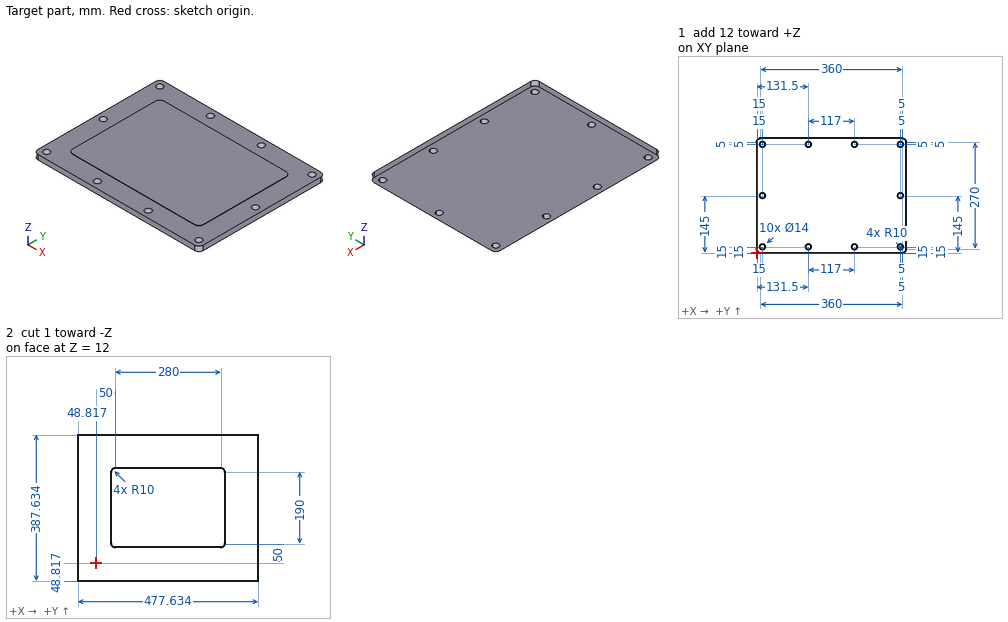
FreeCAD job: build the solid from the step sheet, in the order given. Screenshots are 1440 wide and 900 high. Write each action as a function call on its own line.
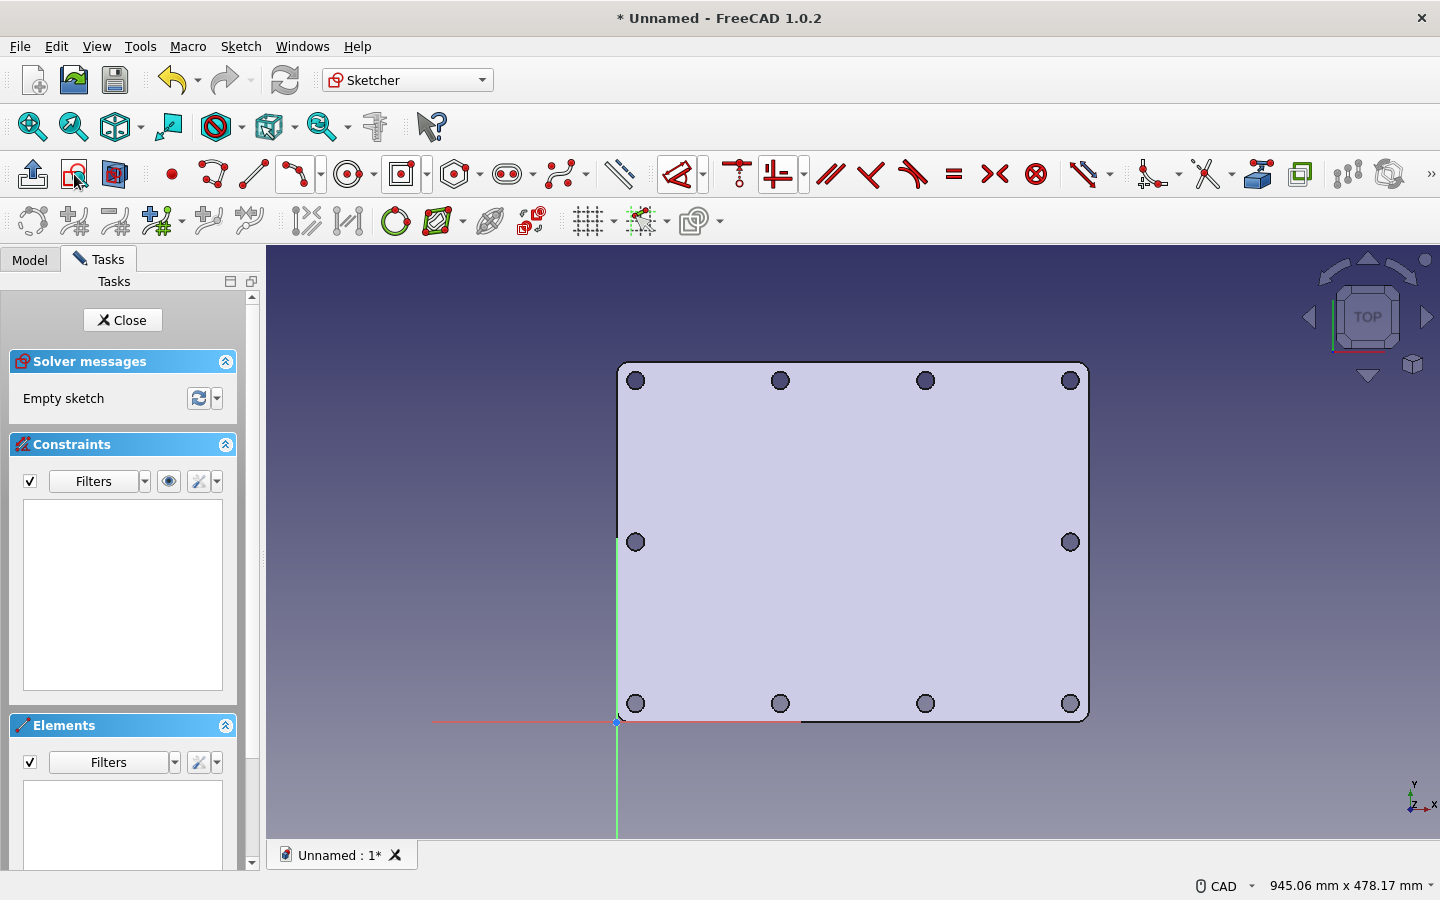
key(g)
key(r)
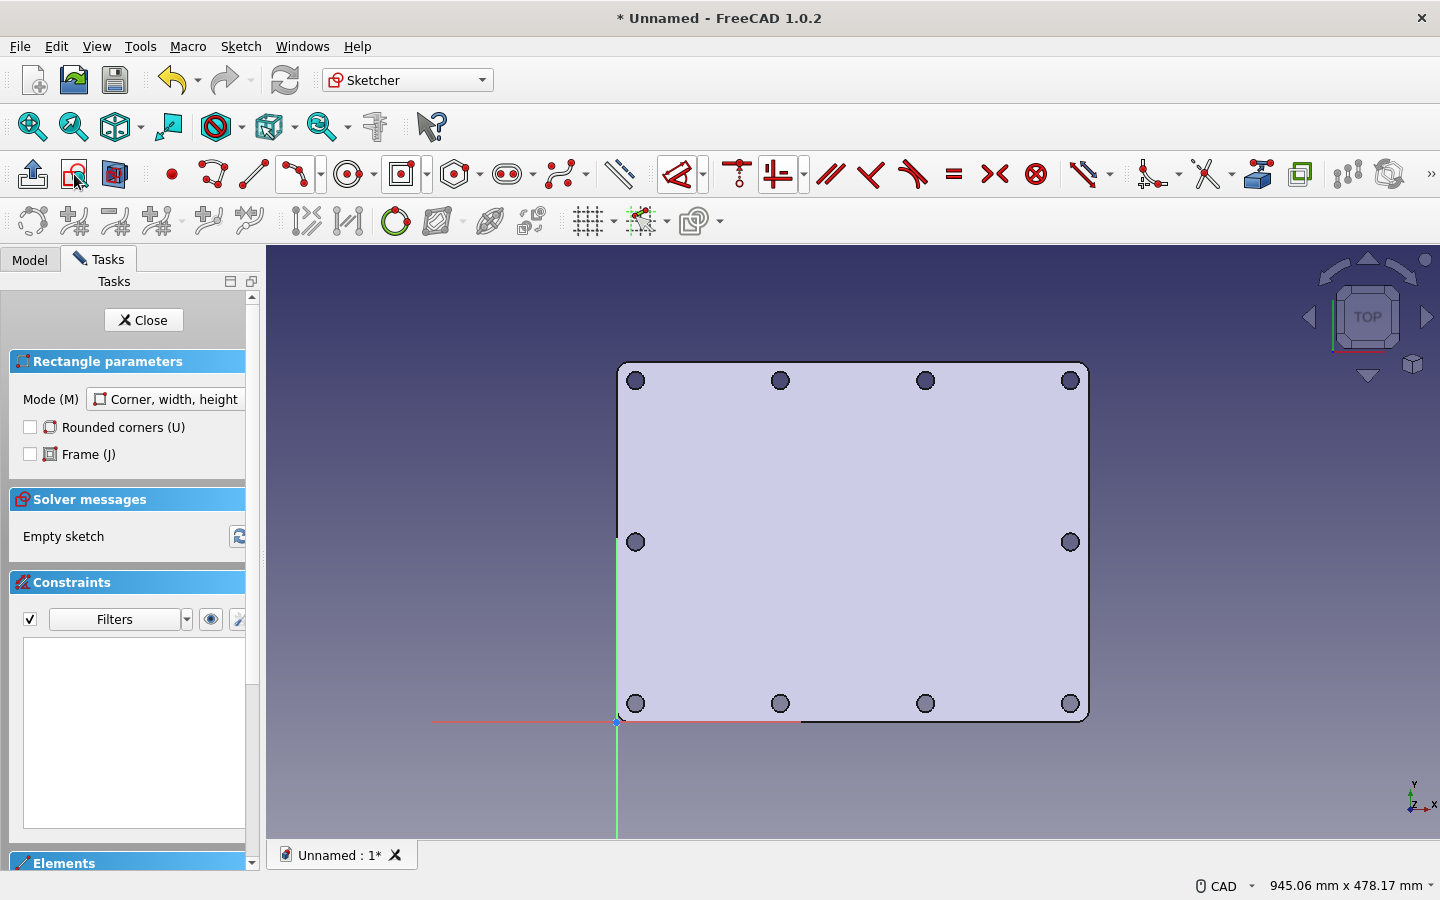
click(556, 301)
click(1150, 783)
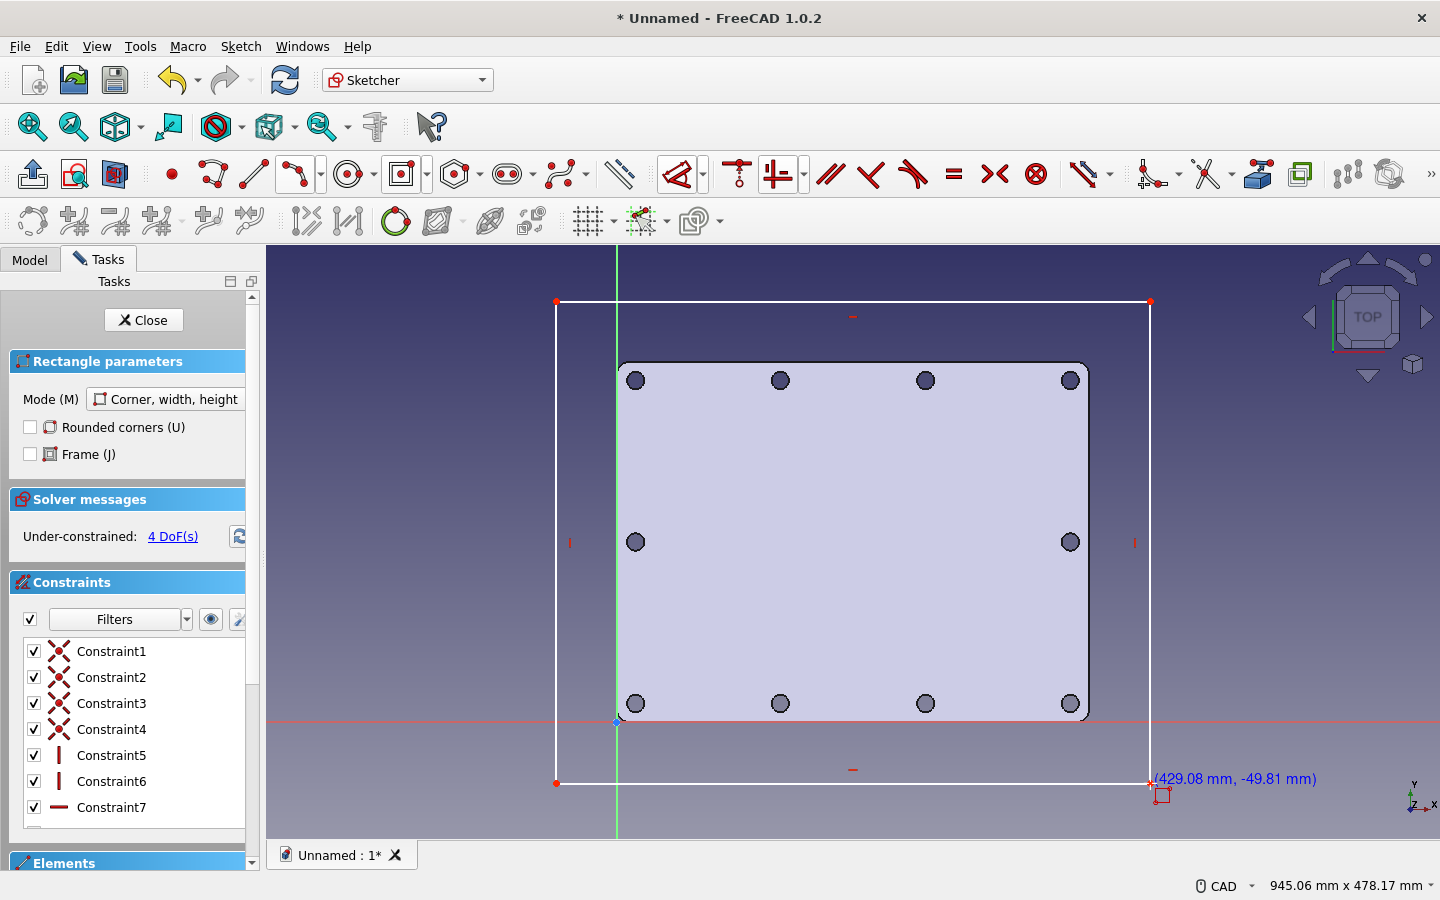
click(254, 174)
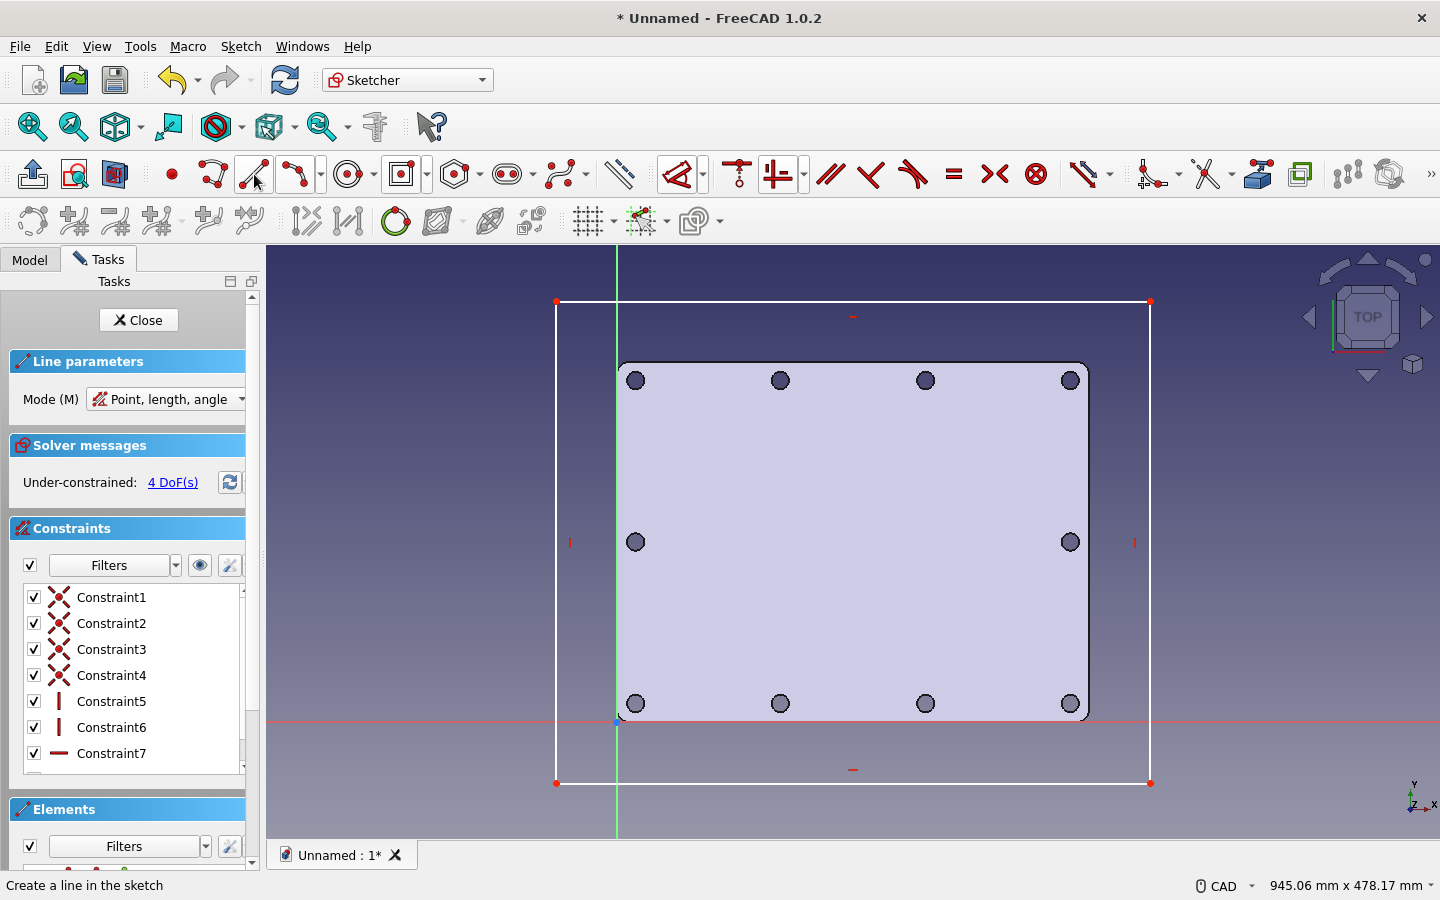
click(679, 412)
click(1027, 412)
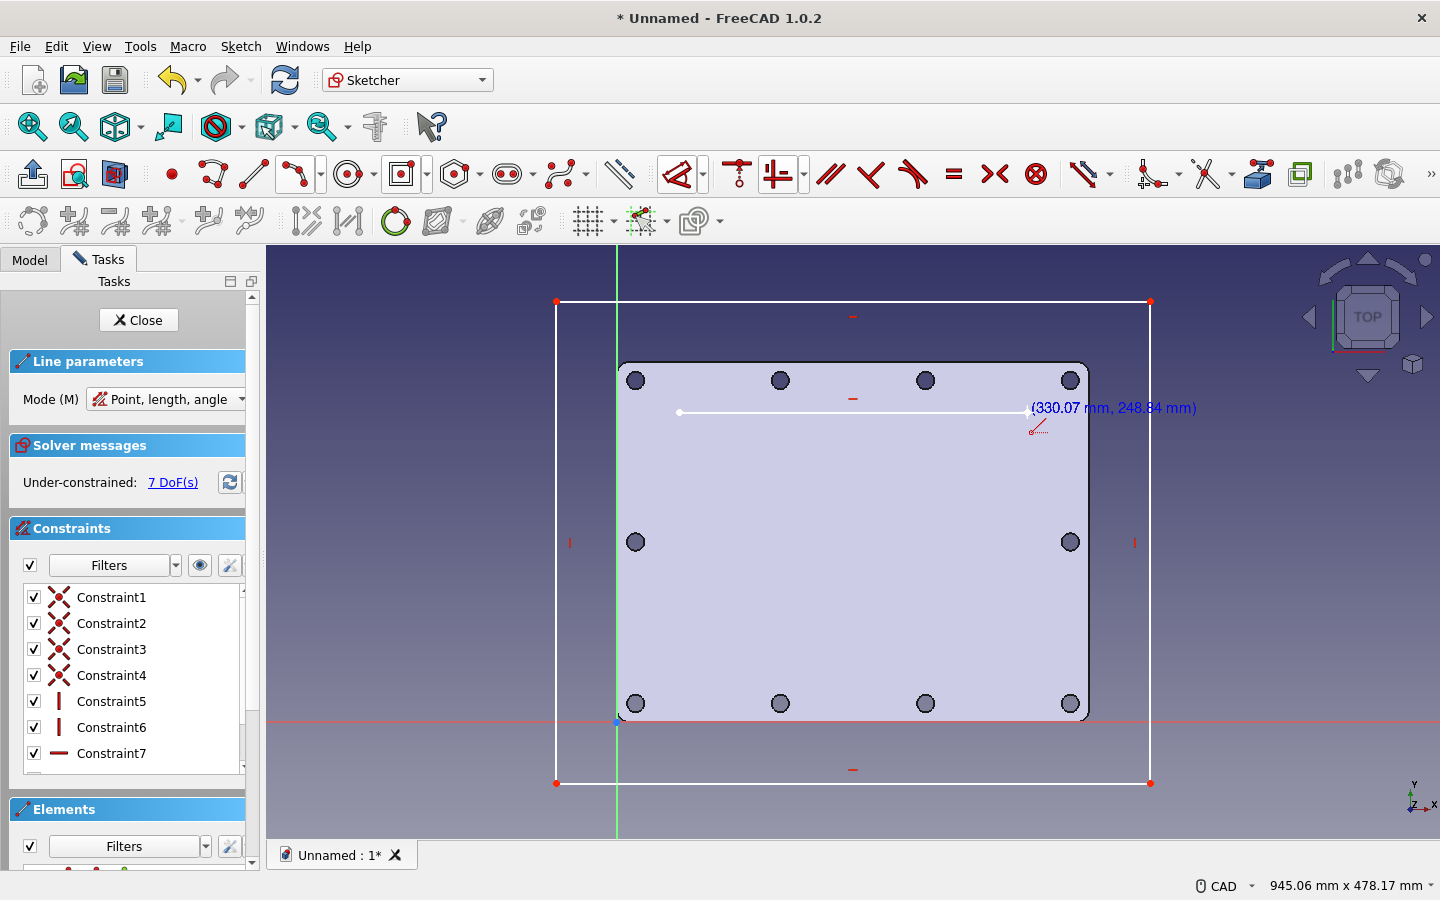
click(1039, 424)
click(1039, 660)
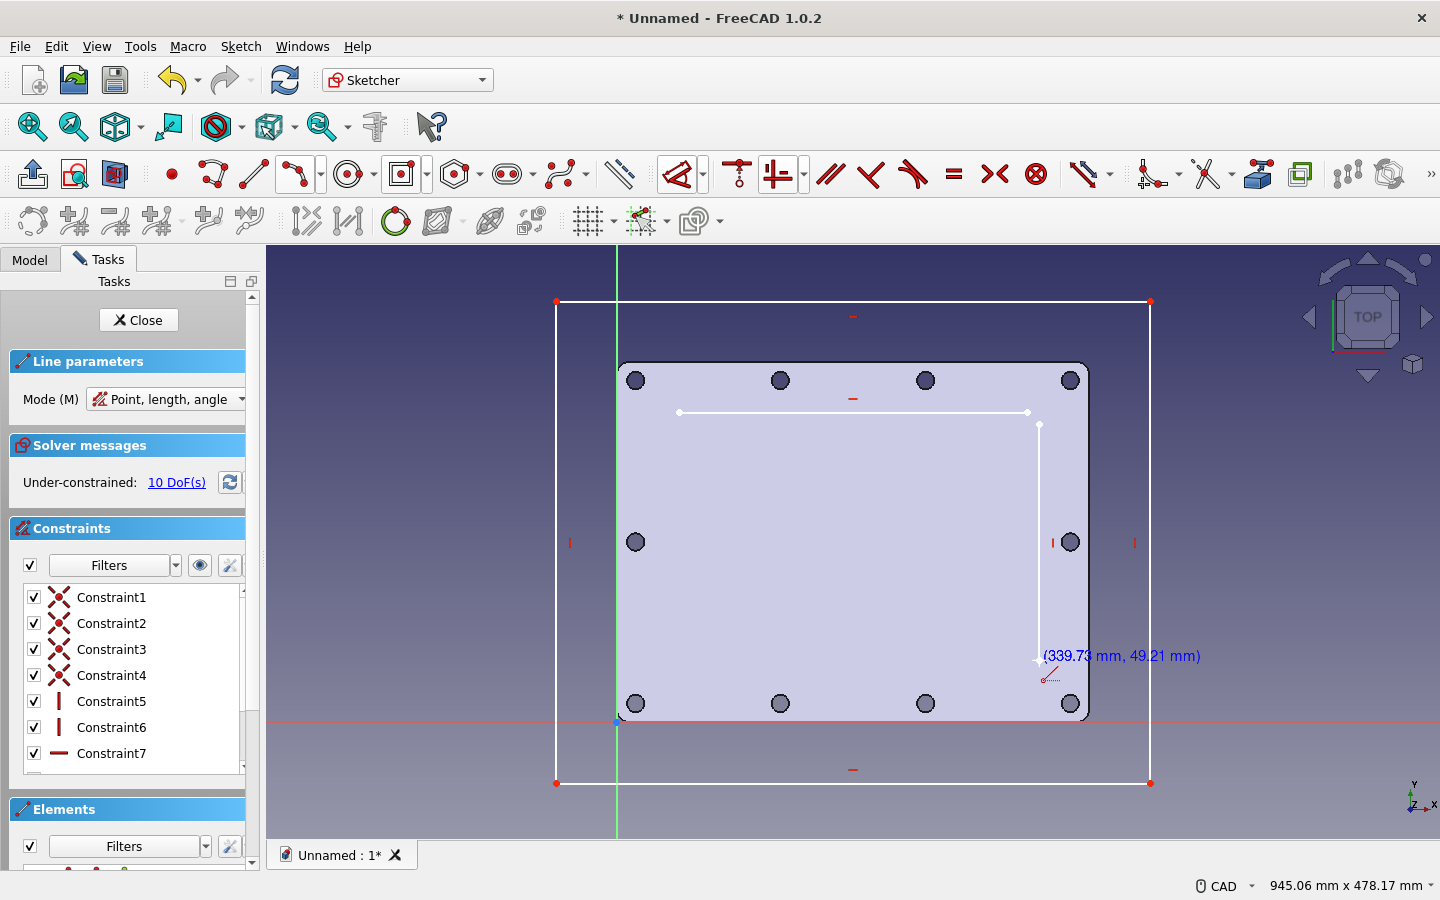
click(1027, 672)
click(679, 672)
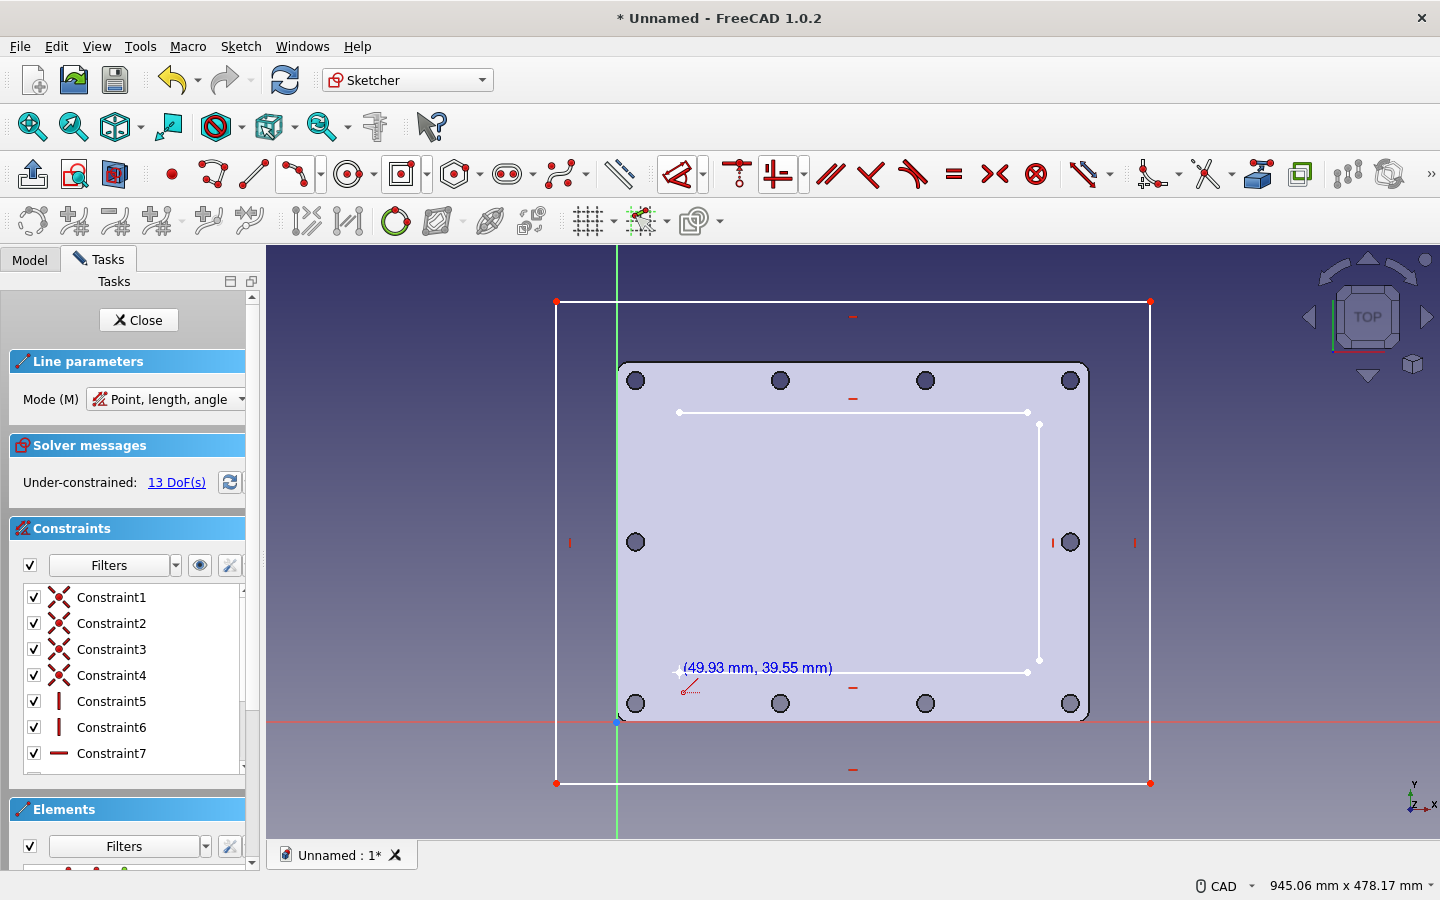
click(667, 660)
click(667, 424)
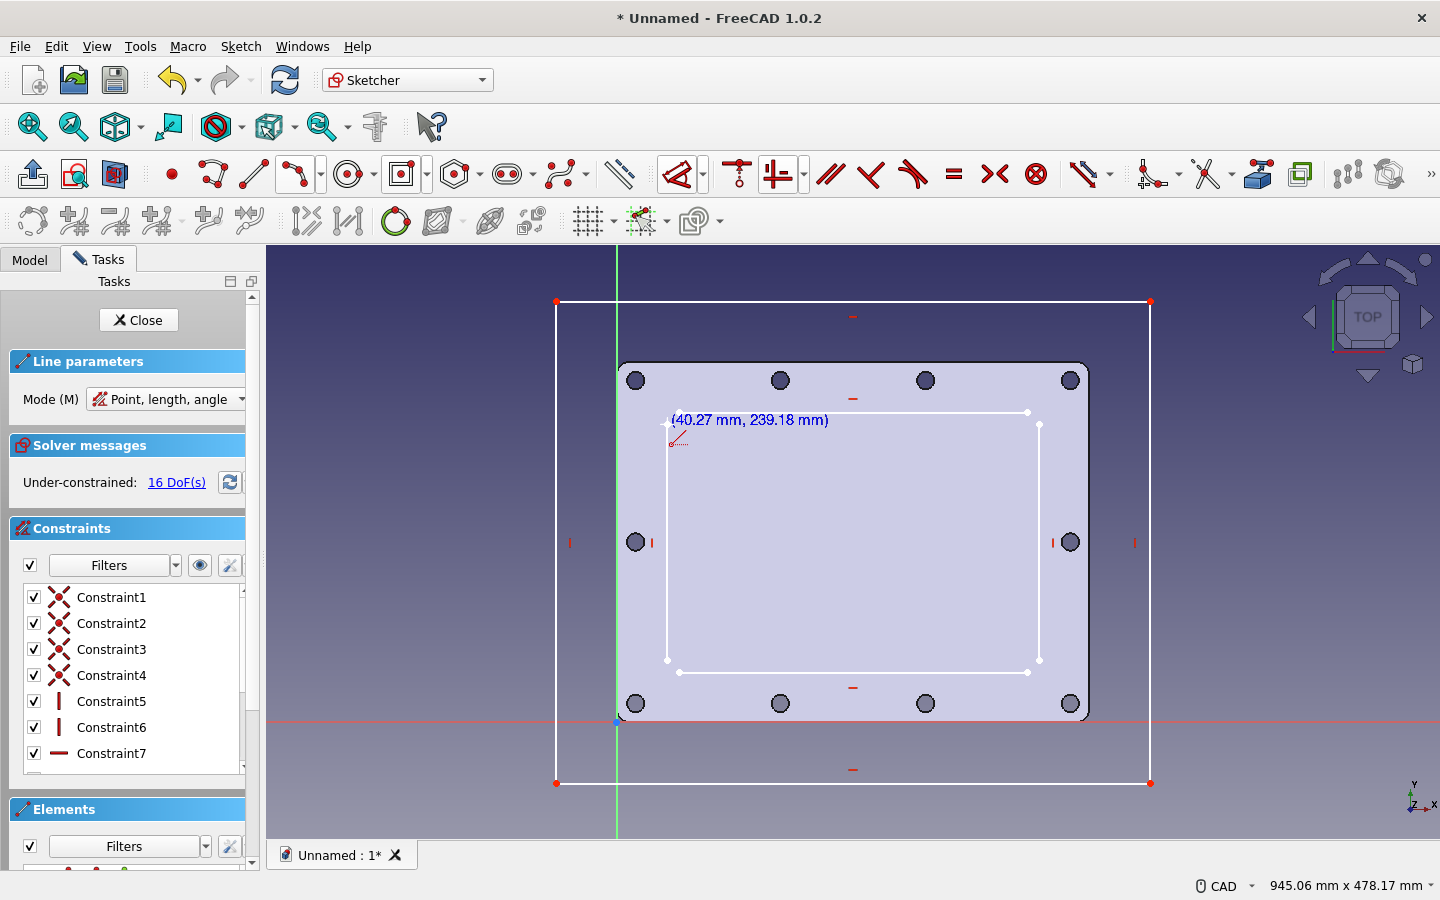
click(294, 174)